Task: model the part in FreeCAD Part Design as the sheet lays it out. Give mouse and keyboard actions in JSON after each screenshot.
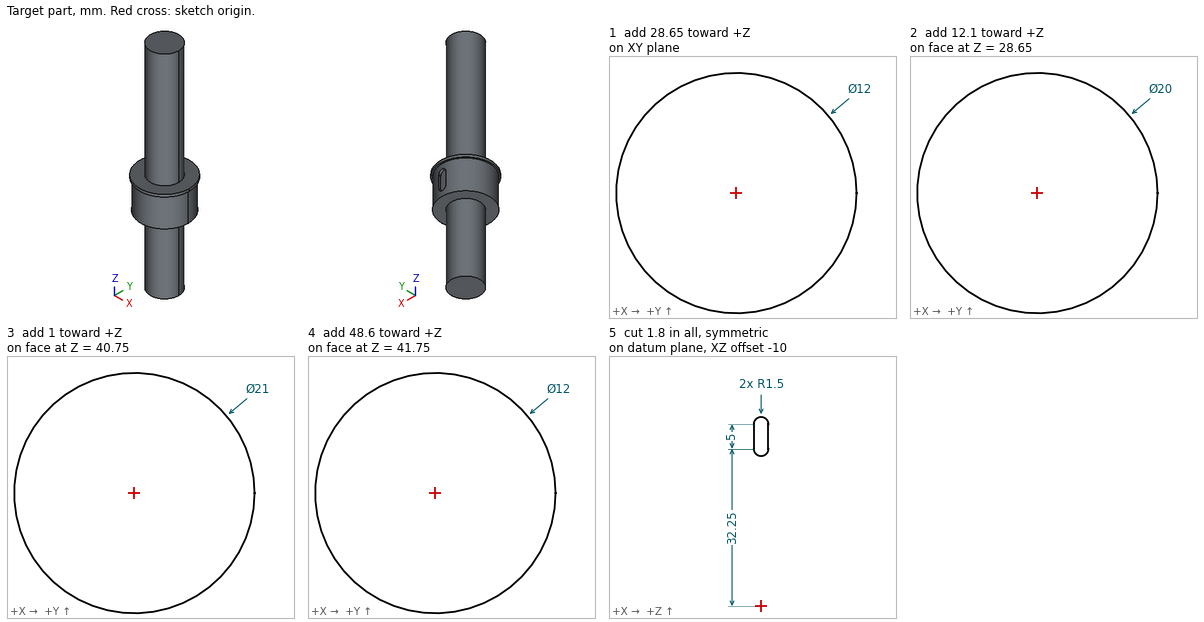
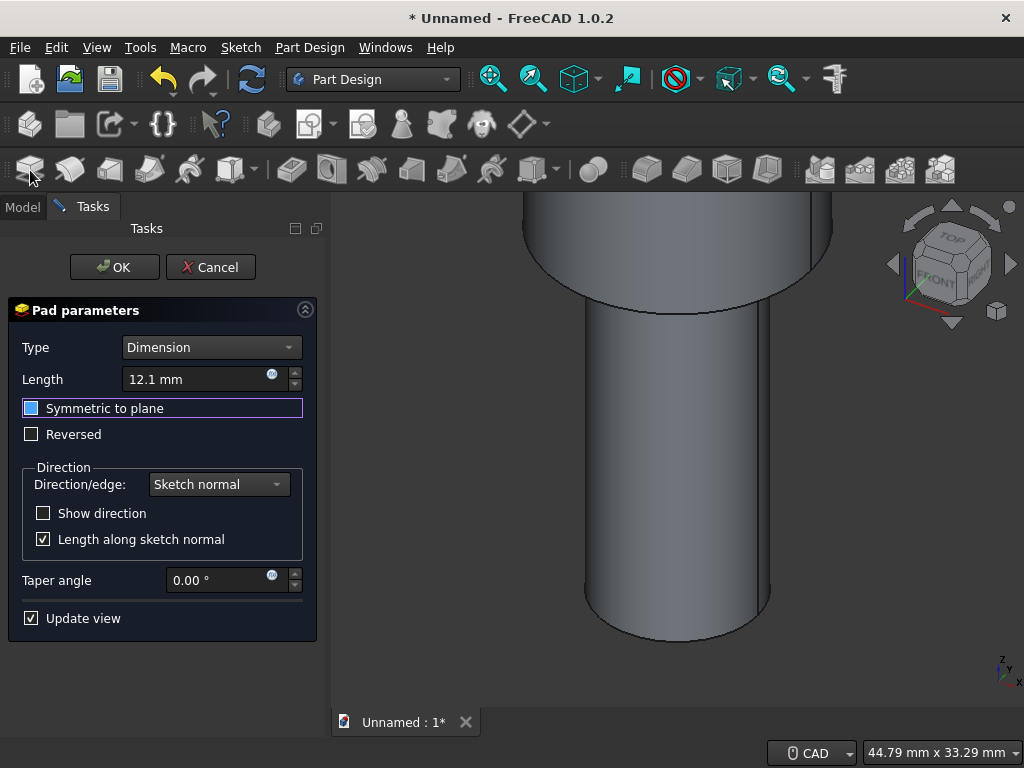
{"action": "left_click", "coordinate": [115, 267]}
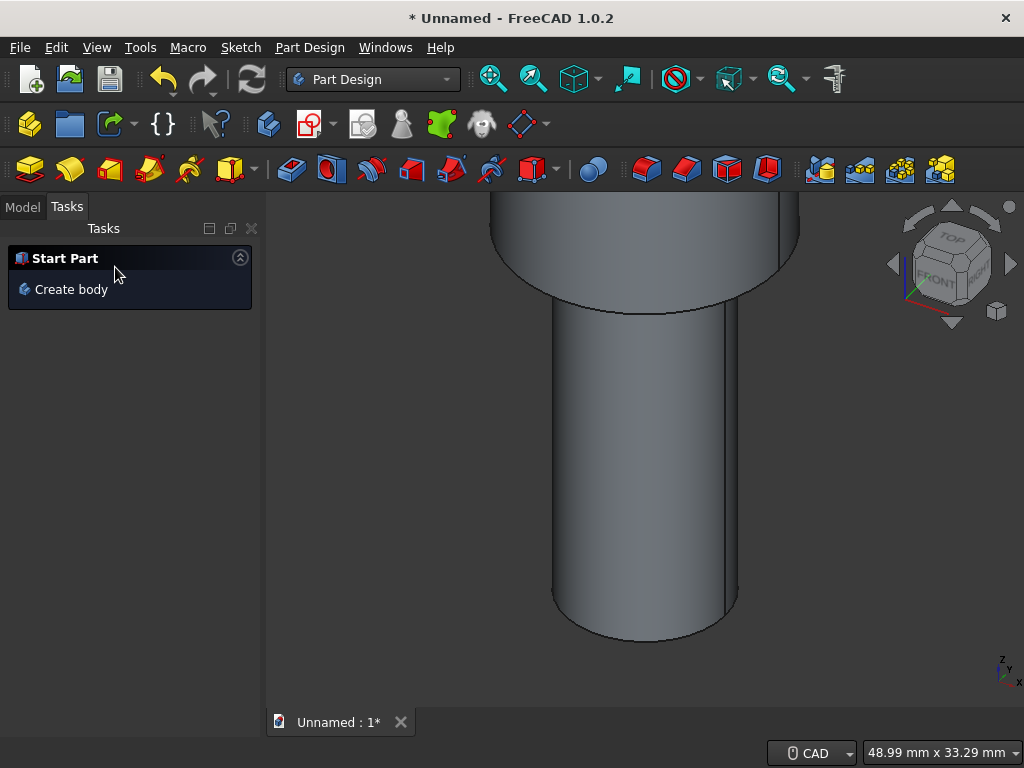
{"action": "left_click", "coordinate": [494, 80]}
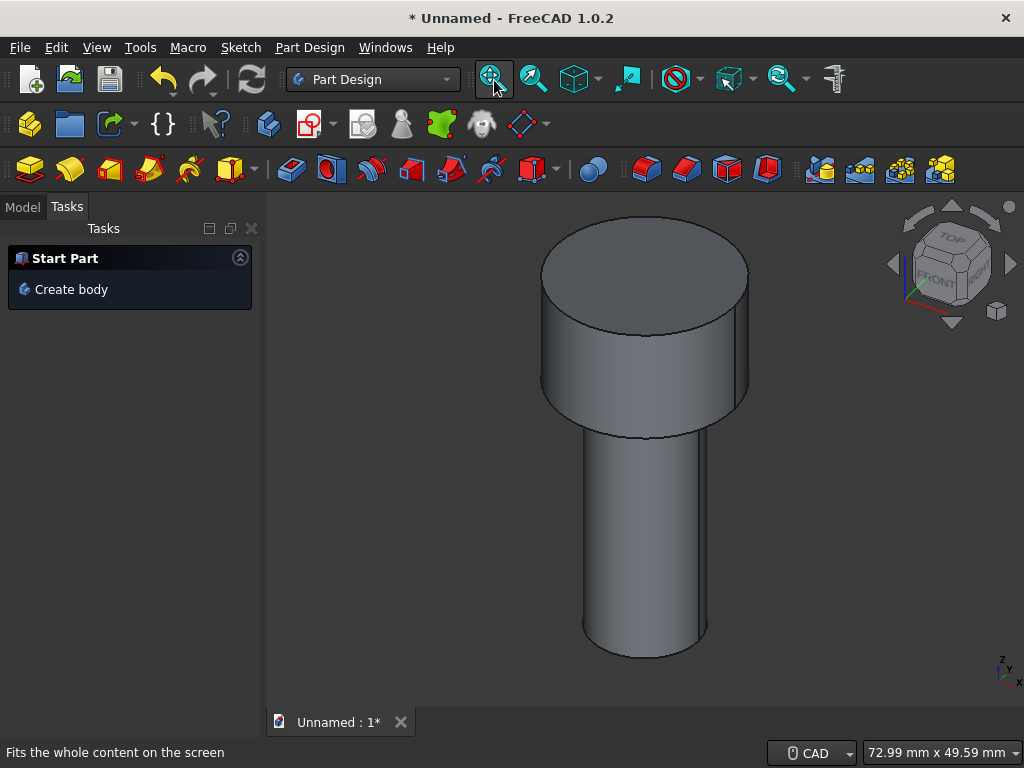
{"action": "left_click", "coordinate": [645, 275]}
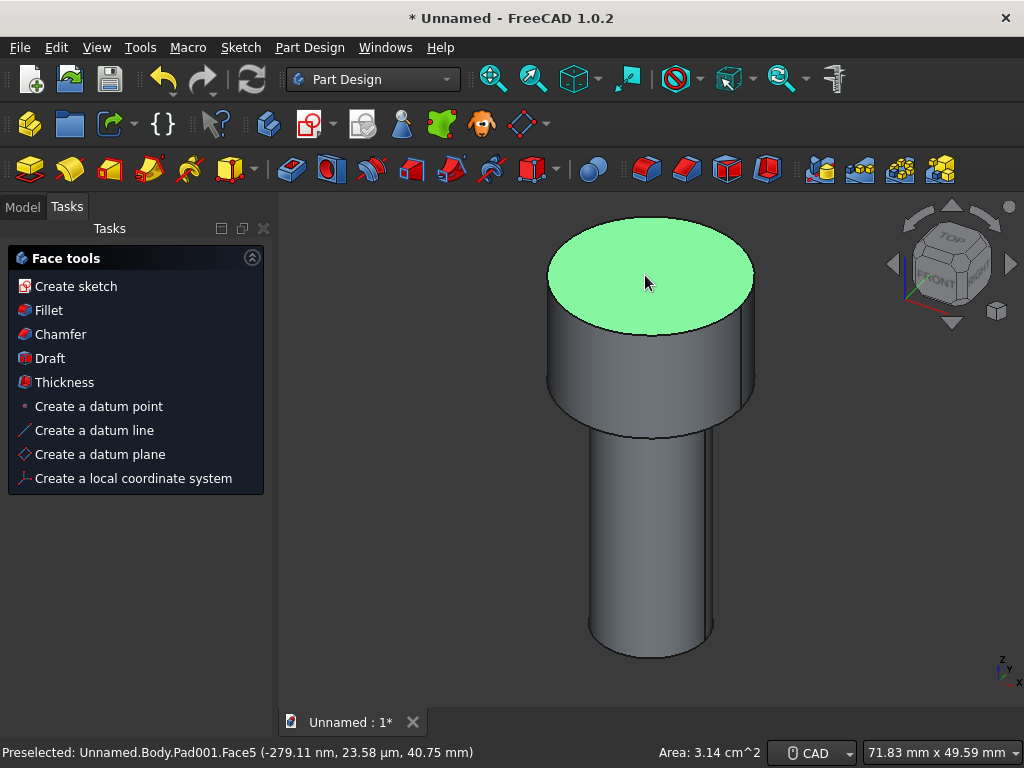
{"action": "left_click", "coordinate": [310, 124]}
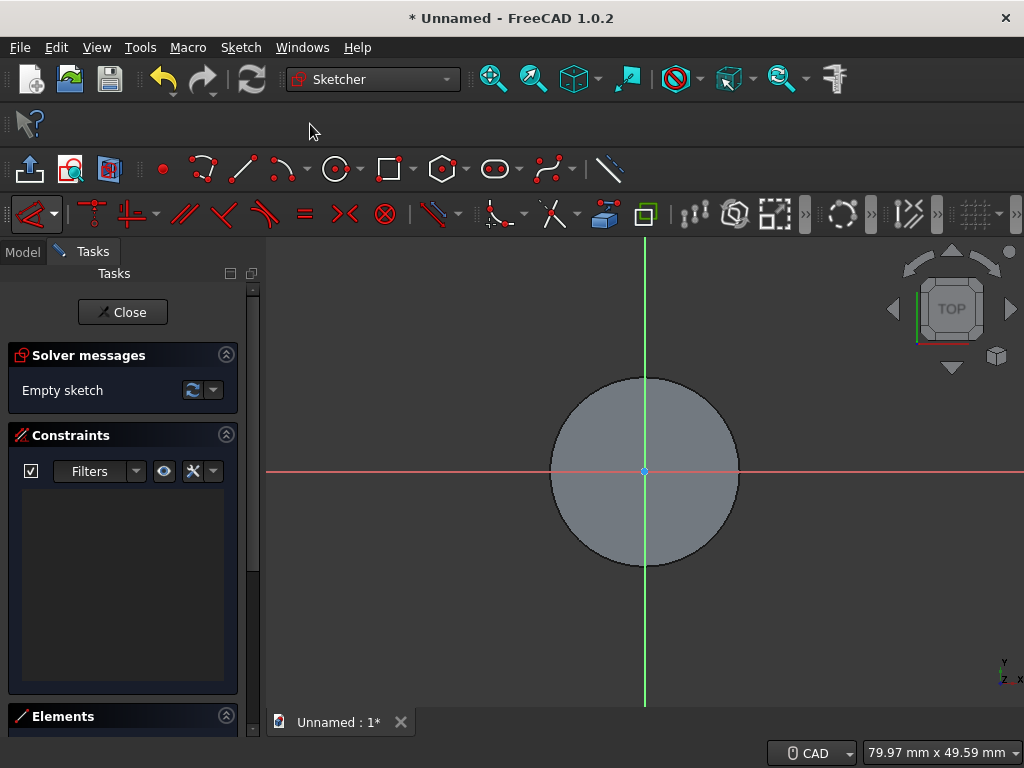
{"action": "scroll", "coordinate": [784, 472], "scroll_direction": "up", "scroll_amount": 2}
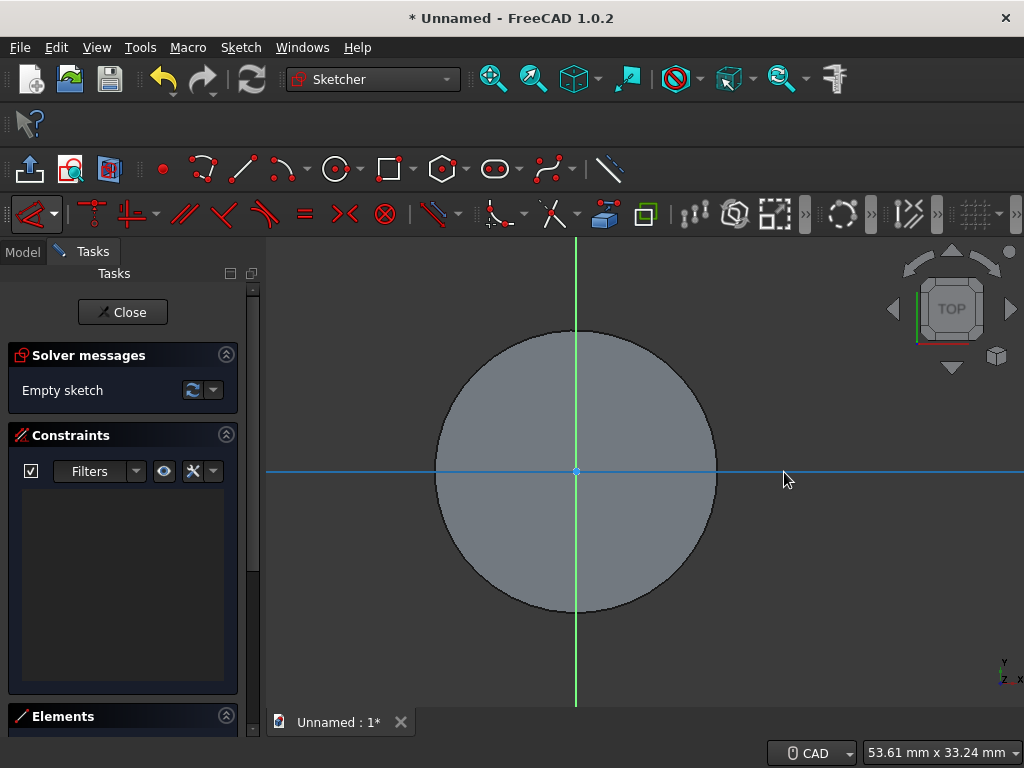
{"action": "left_click", "coordinate": [336, 170]}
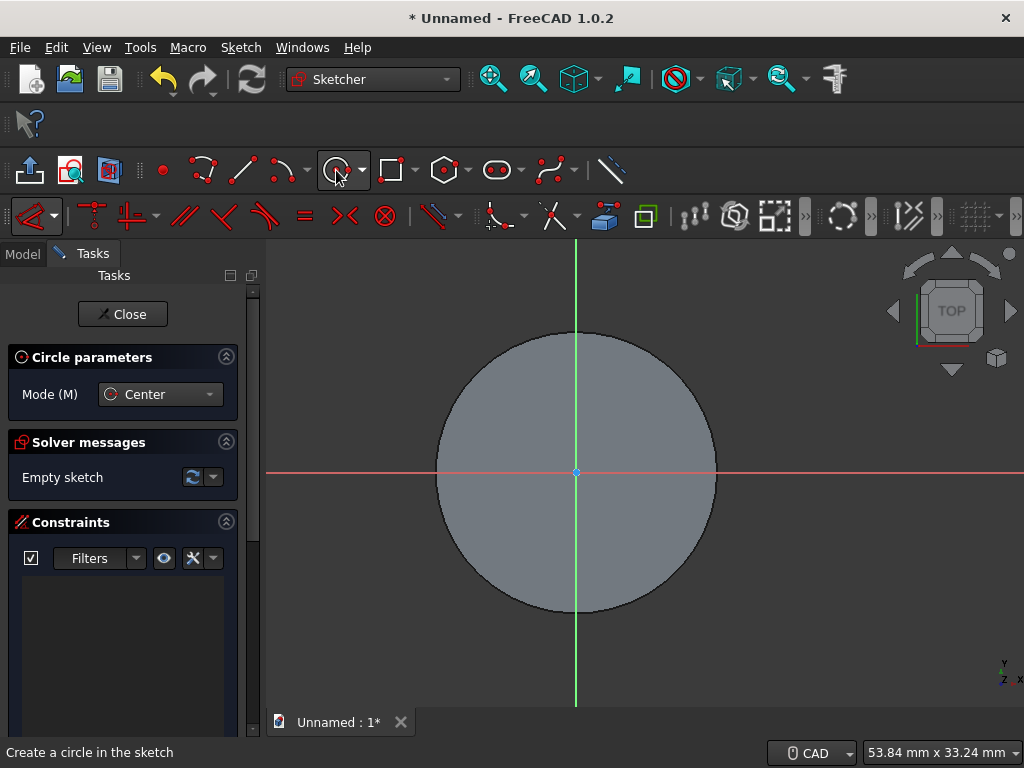
{"action": "left_click", "coordinate": [576, 473]}
{"action": "left_click", "coordinate": [681, 368]}
{"action": "key", "text": "Escape"}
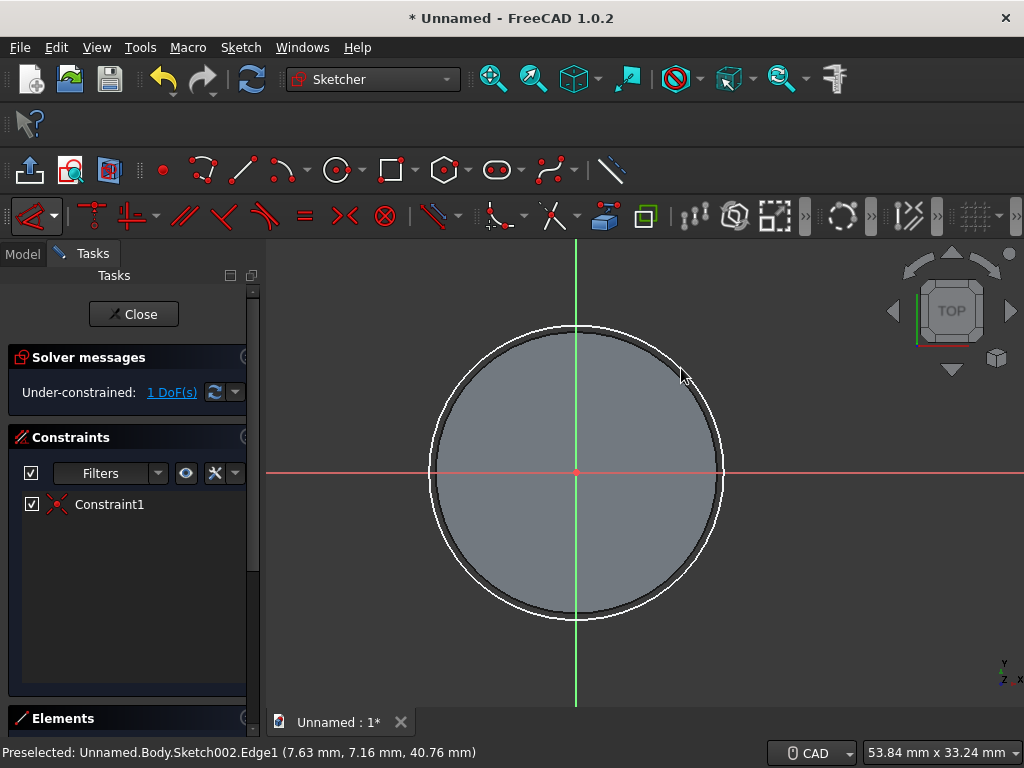
{"action": "left_click", "coordinate": [680, 368]}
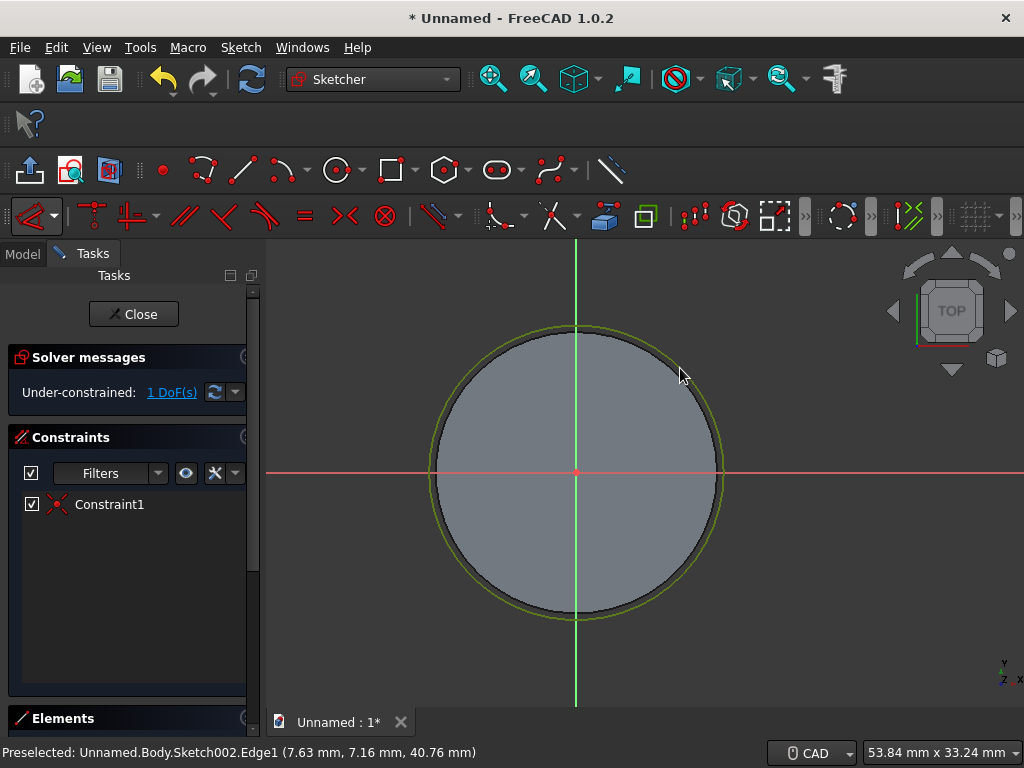
{"action": "key", "text": "k o"}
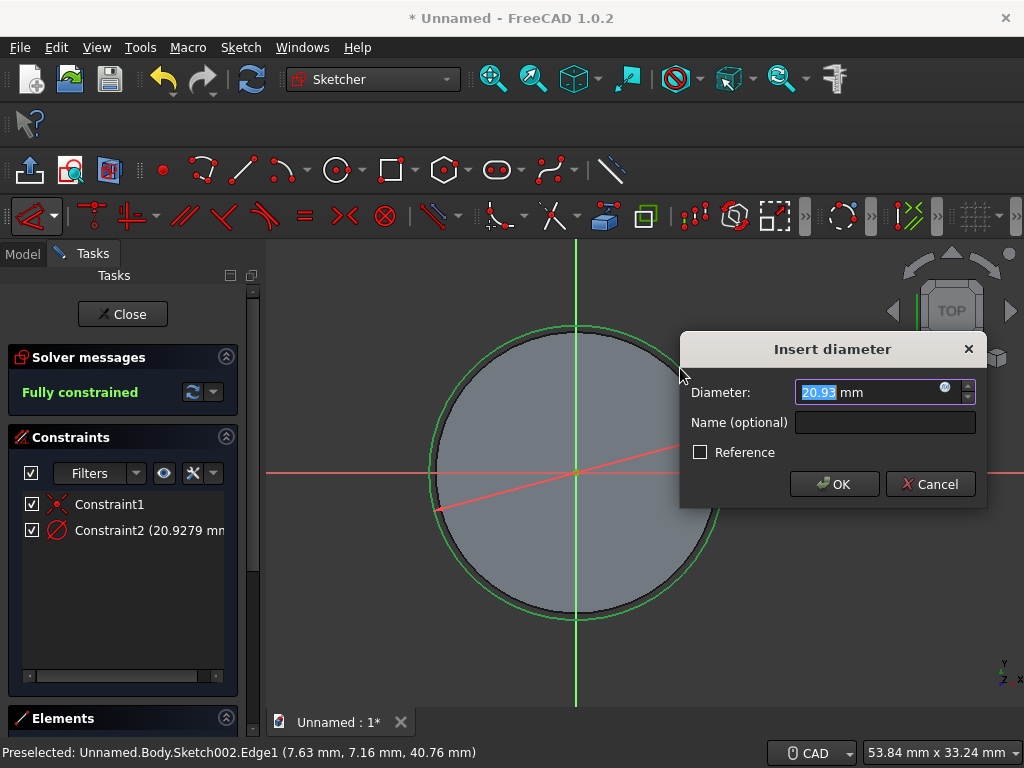
{"action": "type", "text": "21"}
{"action": "key", "text": "Return"}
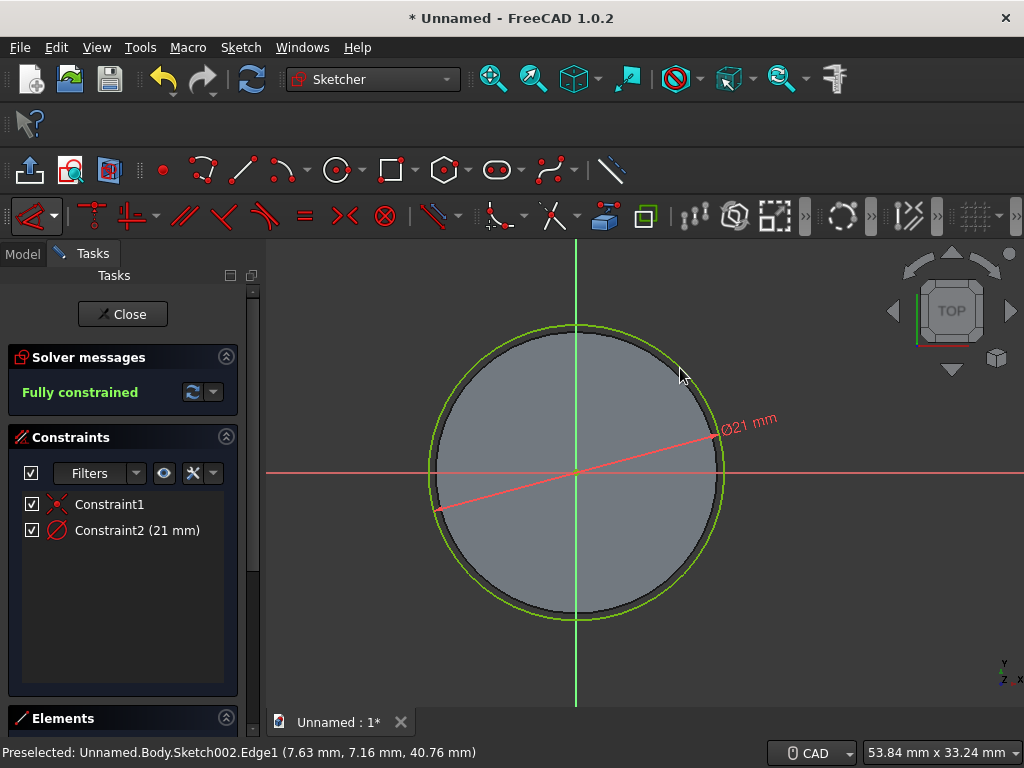
{"action": "left_click", "coordinate": [123, 314]}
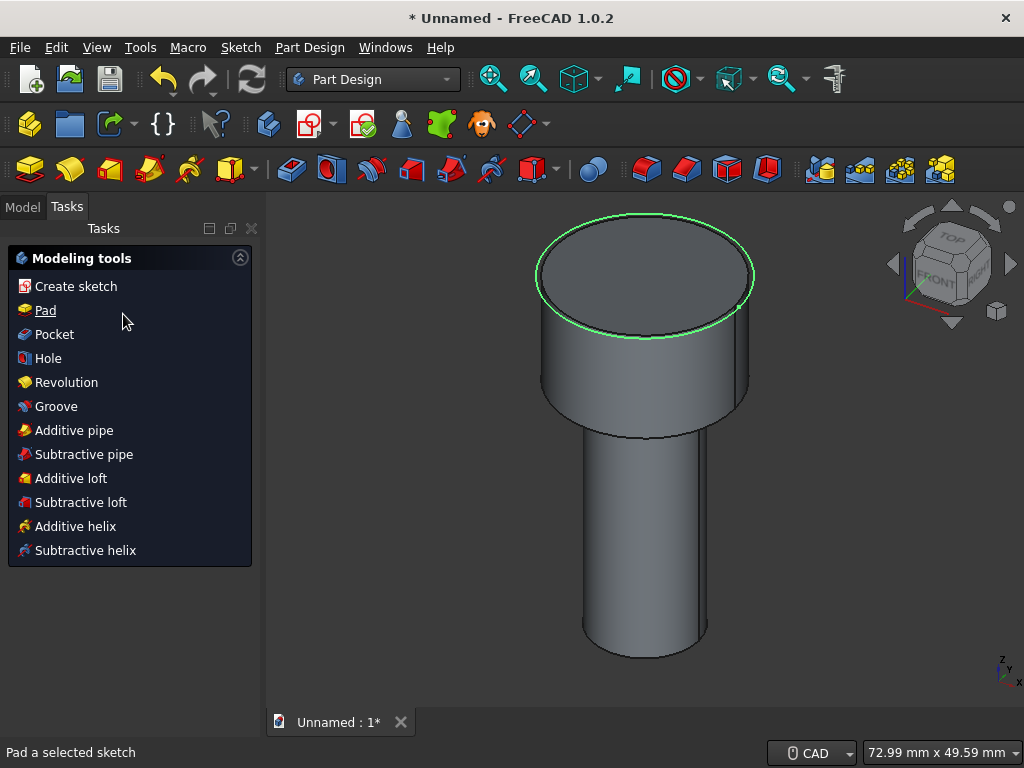
{"action": "left_click", "coordinate": [30, 170]}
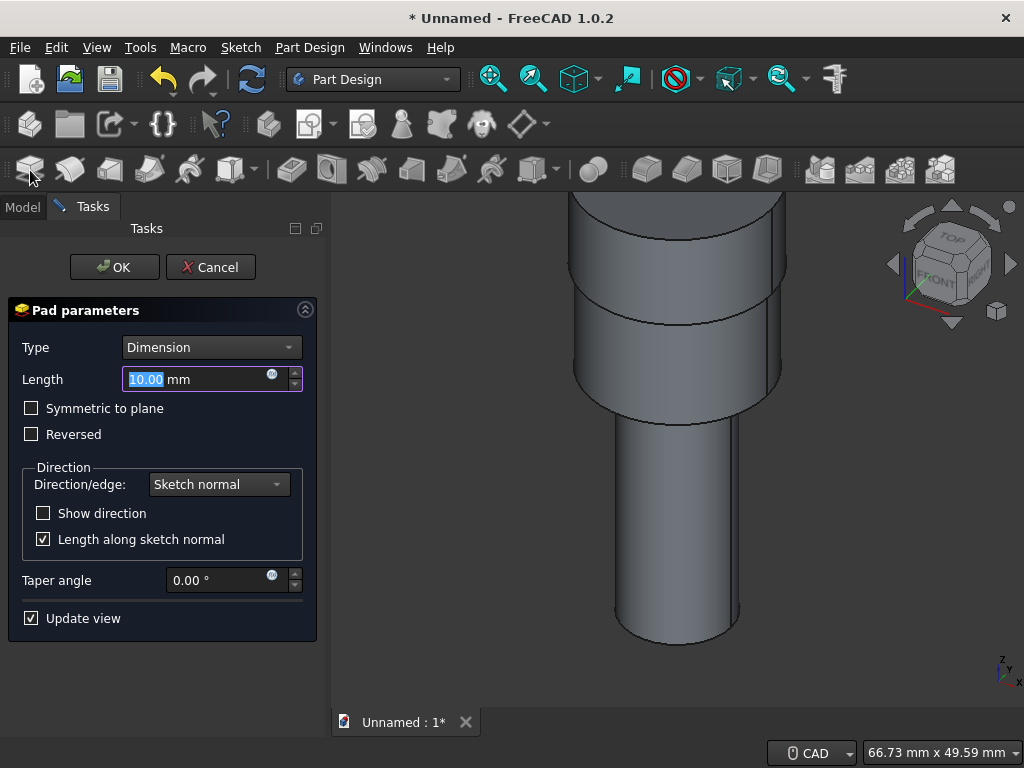
{"action": "type", "text": "1"}
{"action": "key", "text": "Tab"}